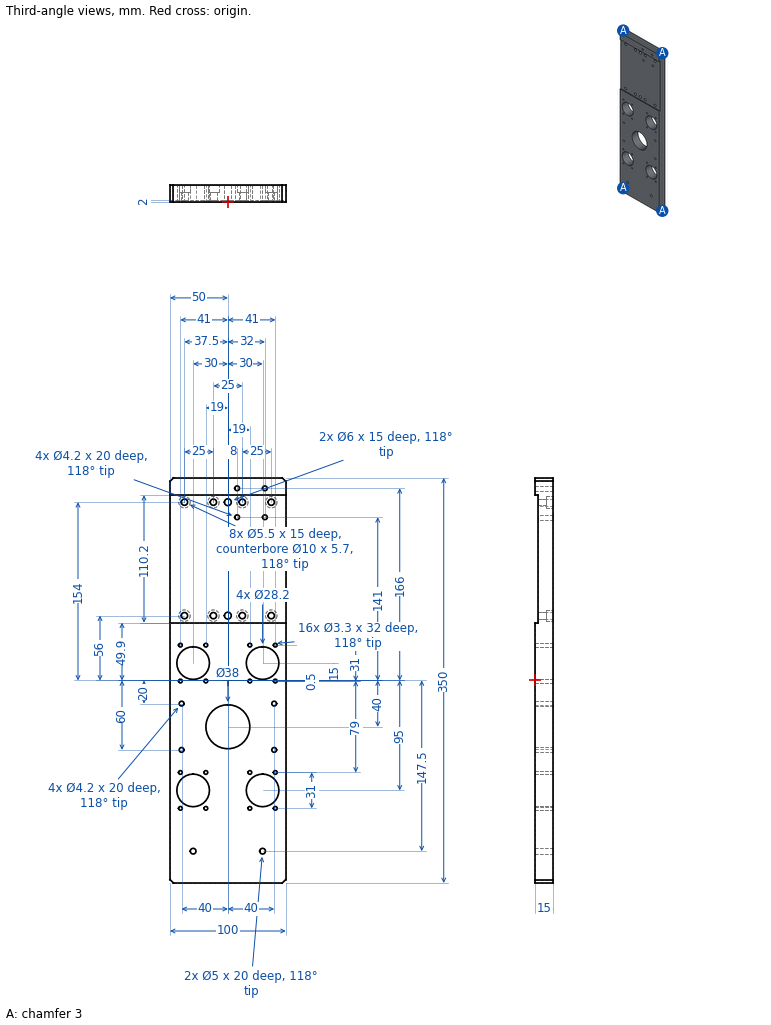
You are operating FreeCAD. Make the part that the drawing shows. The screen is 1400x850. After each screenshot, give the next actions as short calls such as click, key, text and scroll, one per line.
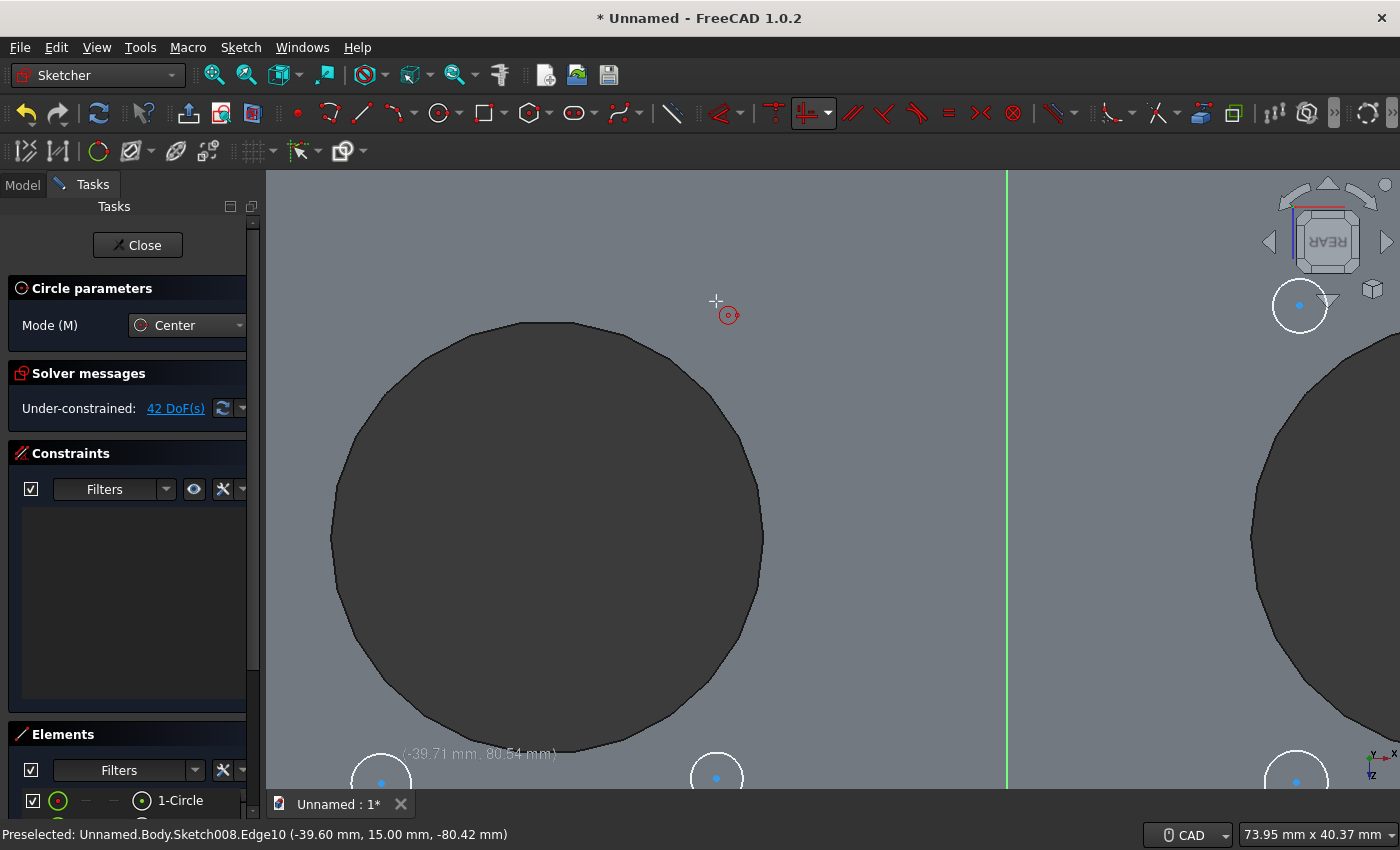
scroll(716, 301, down, 9)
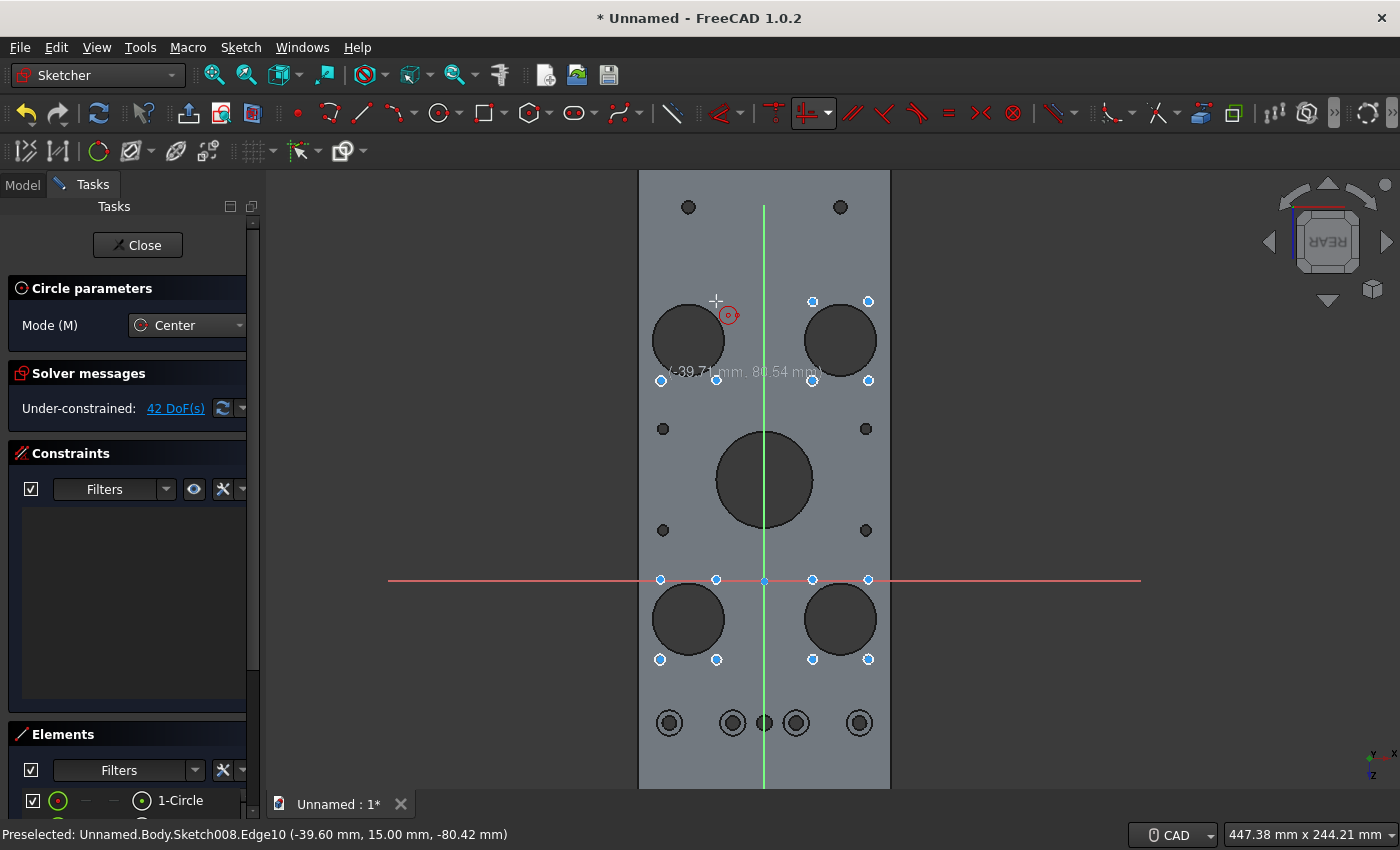
click(716, 301)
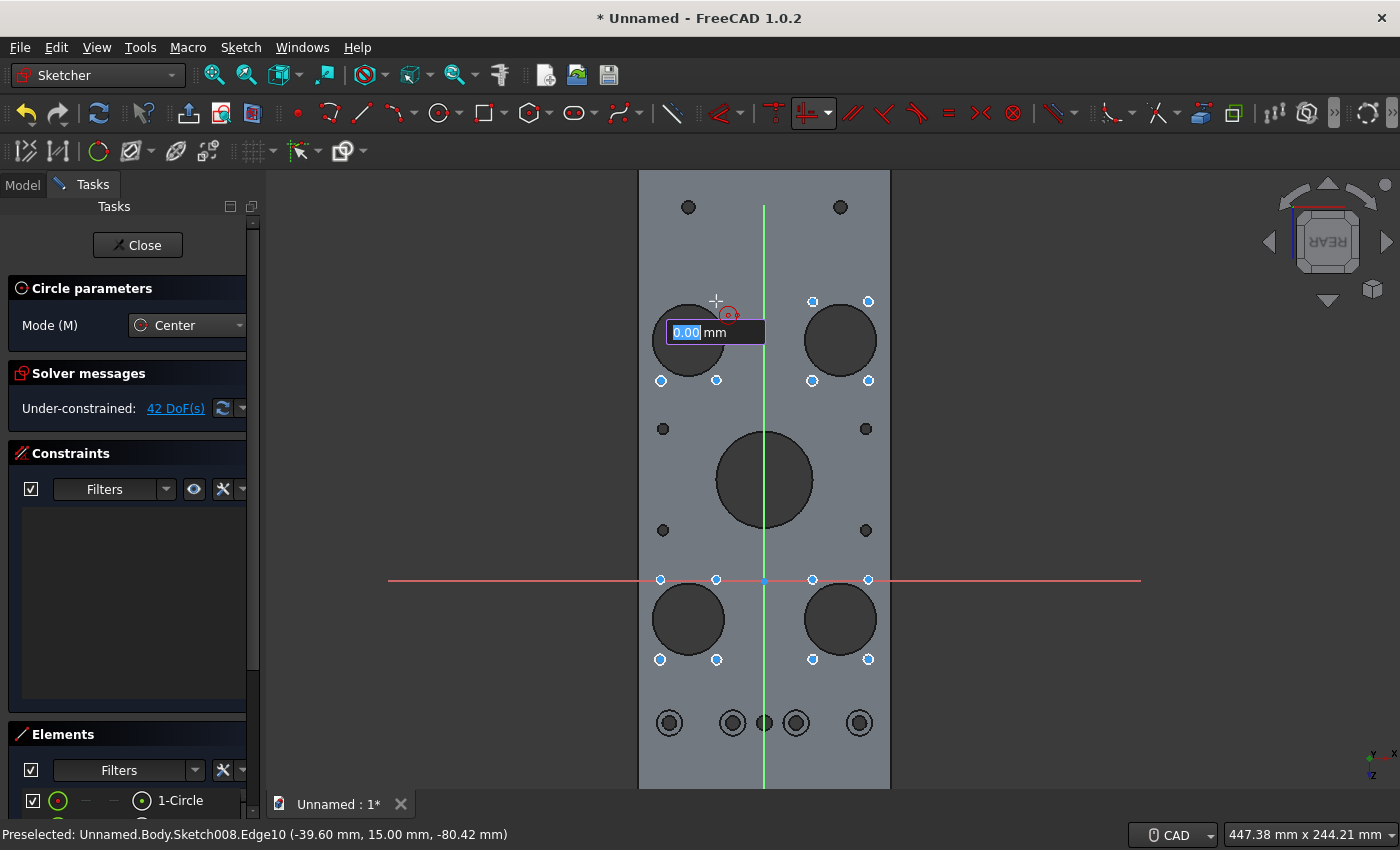
scroll(719, 298, up, 7)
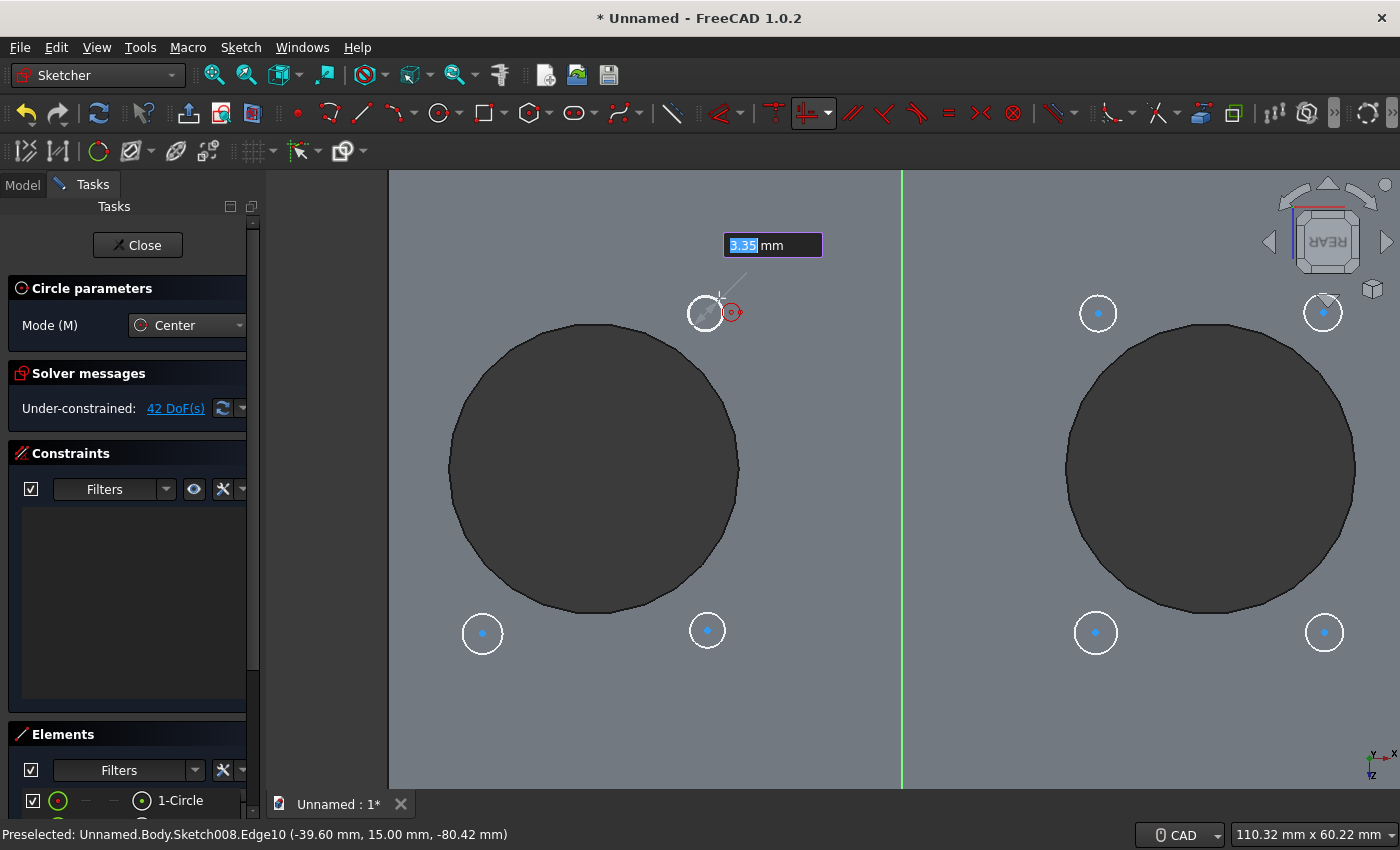
click(719, 298)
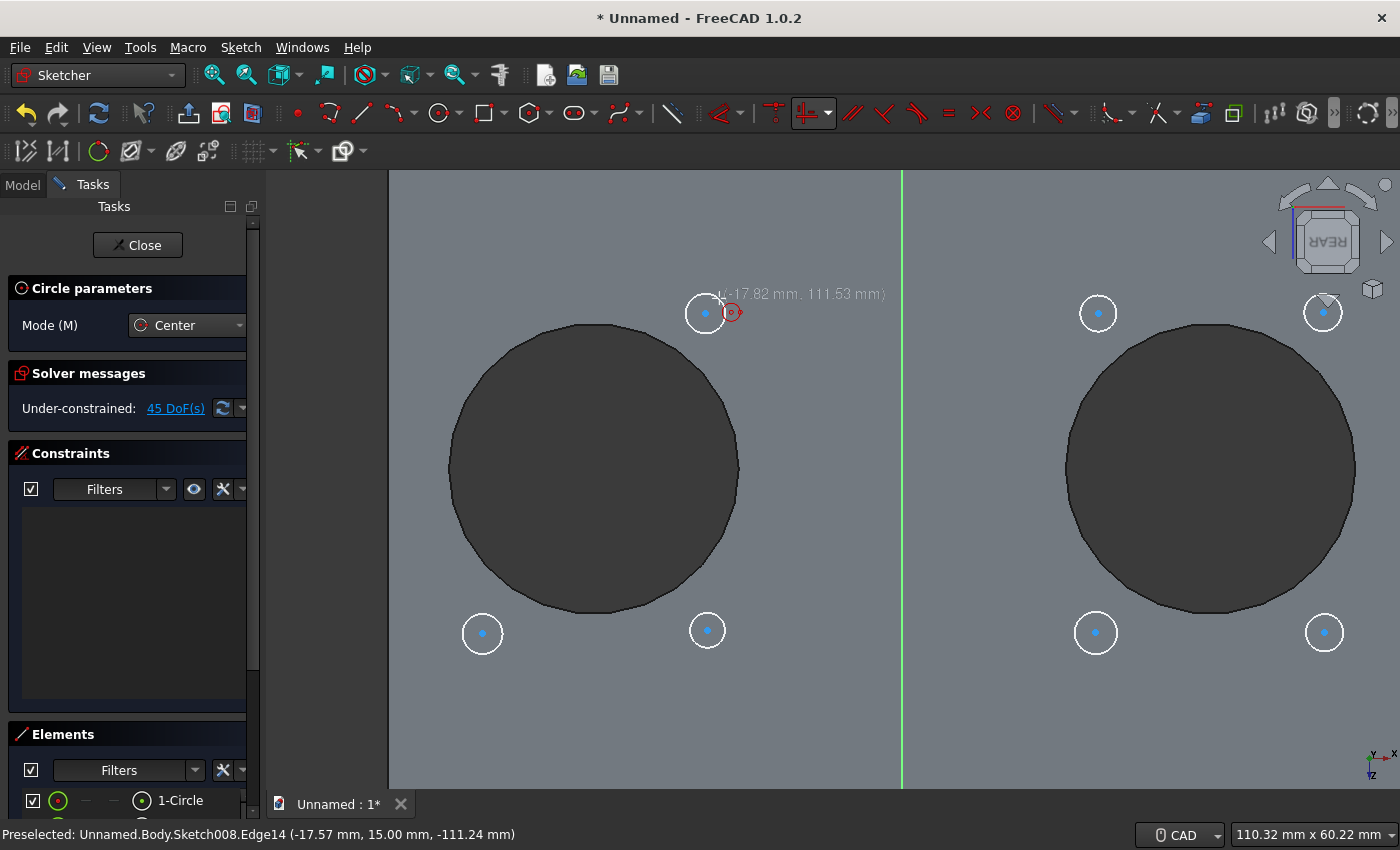
scroll(481, 310, up, 2)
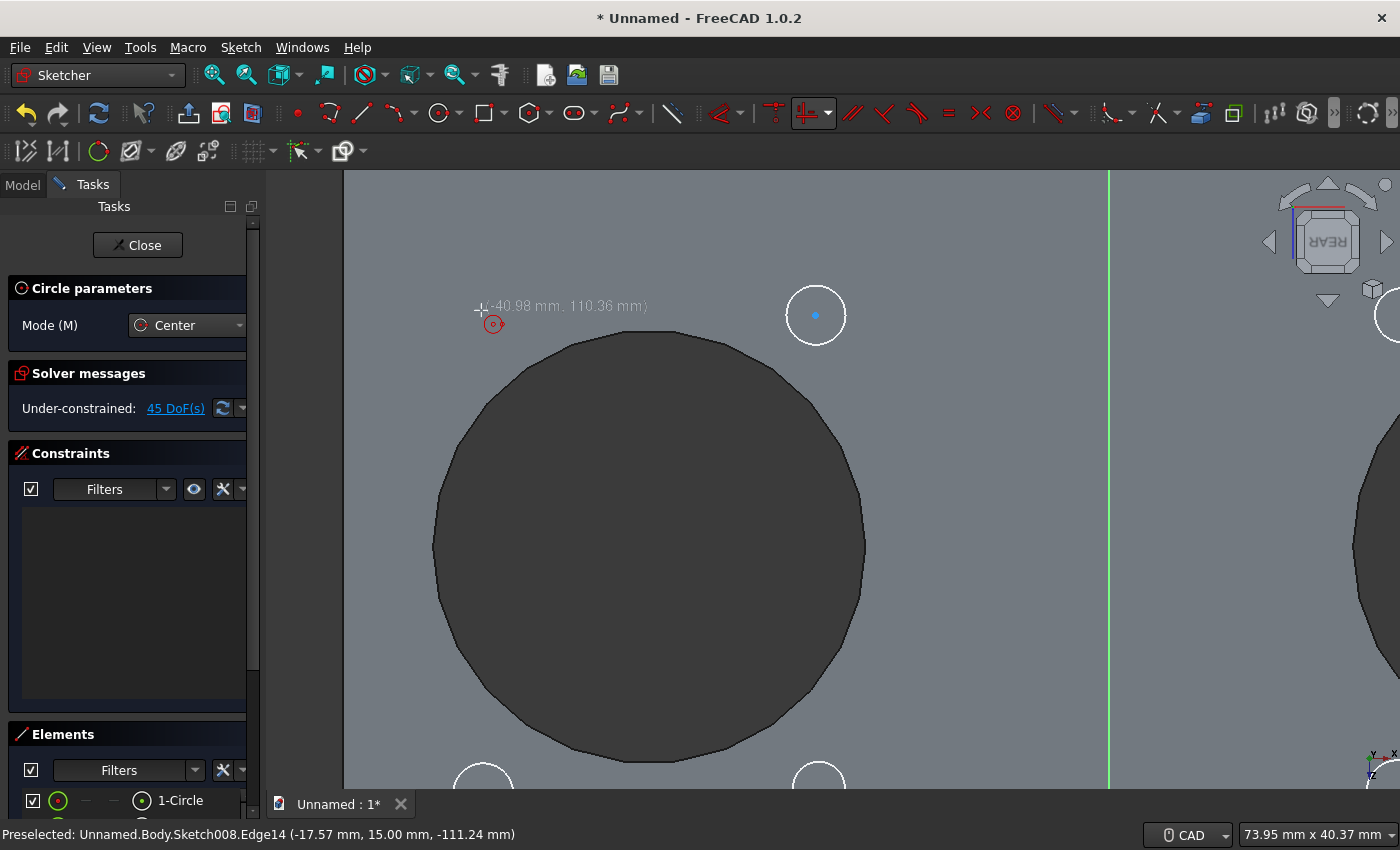
scroll(696, 299, down, 9)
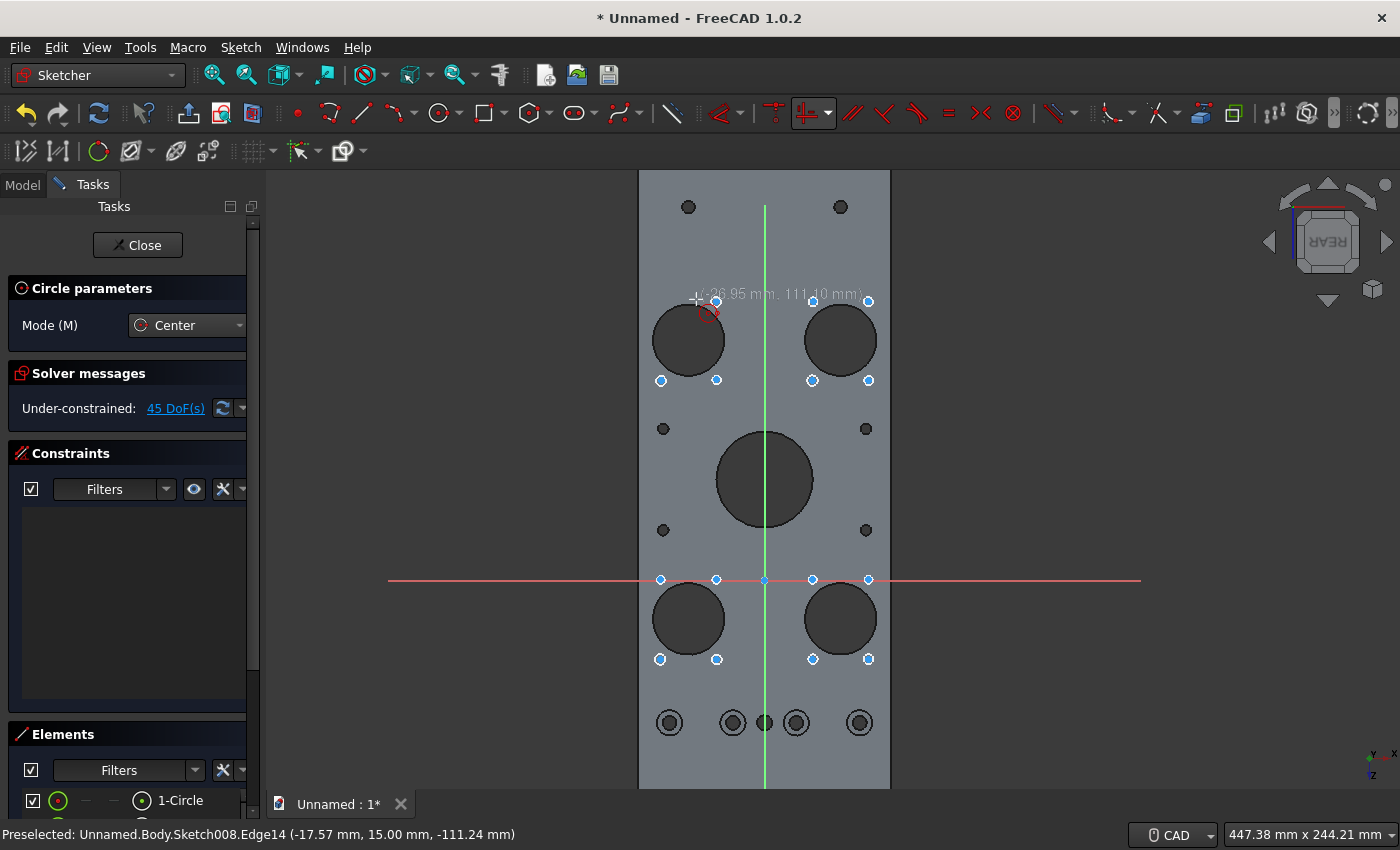
click(661, 301)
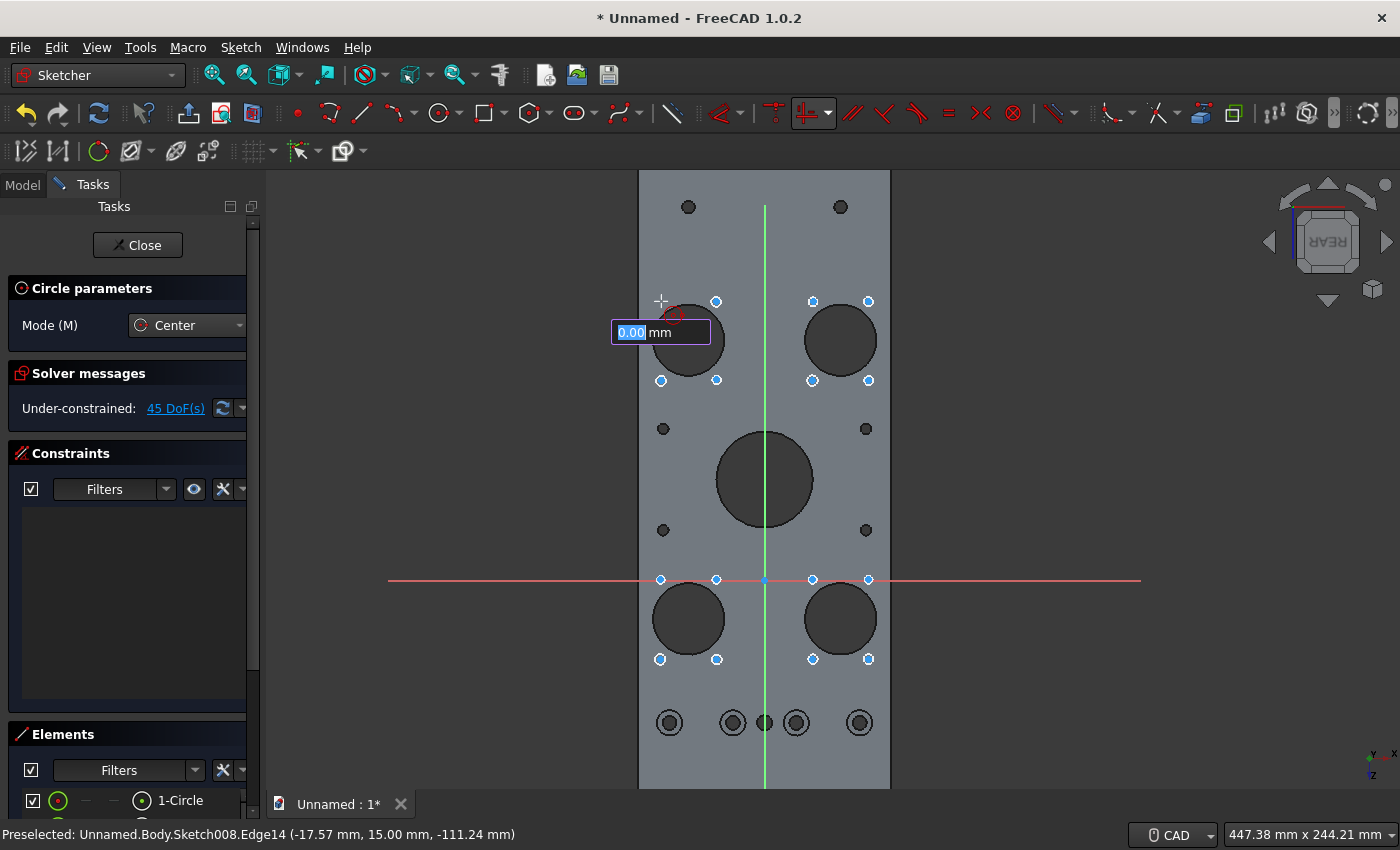
scroll(664, 298, up, 7)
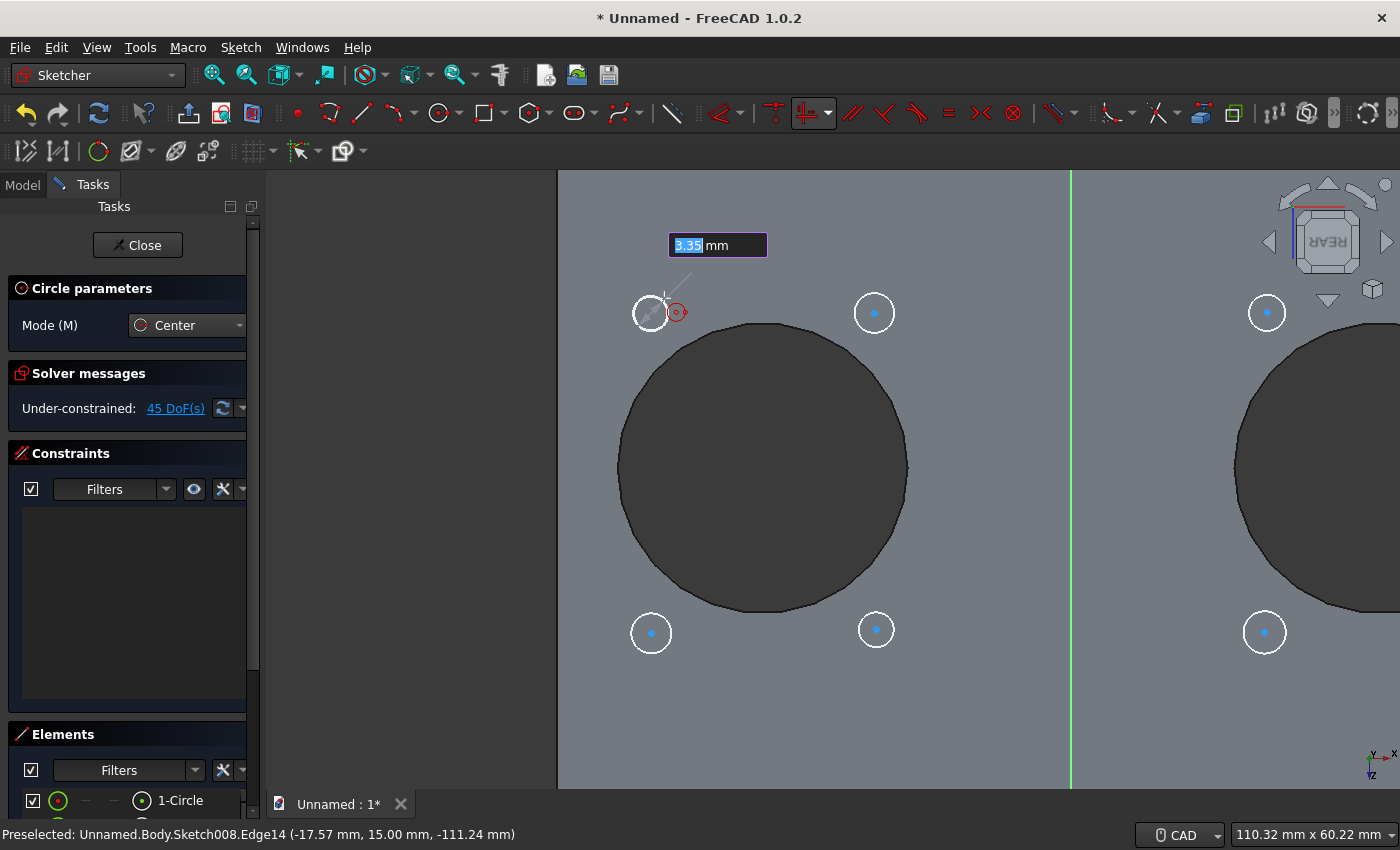
click(662, 297)
key(Escape)